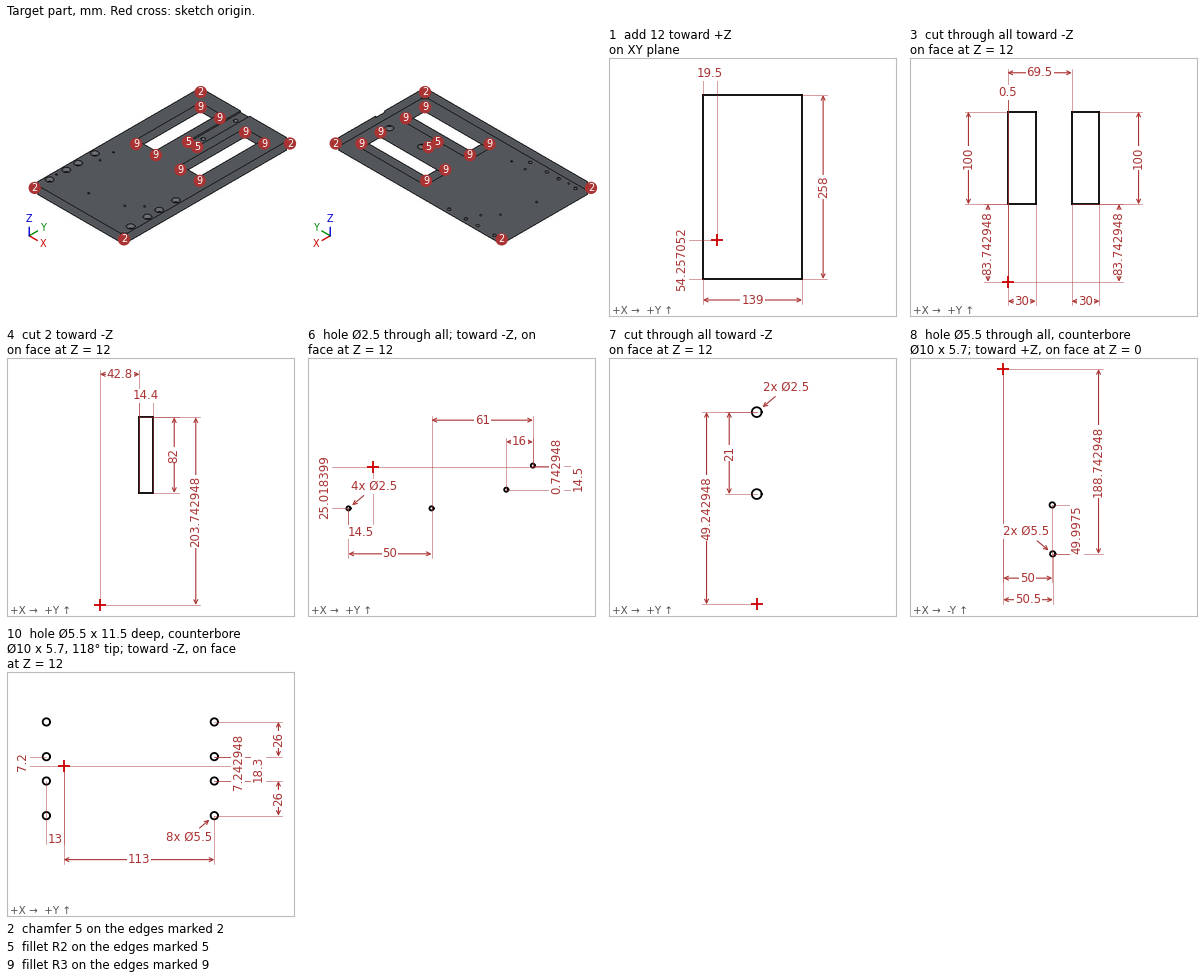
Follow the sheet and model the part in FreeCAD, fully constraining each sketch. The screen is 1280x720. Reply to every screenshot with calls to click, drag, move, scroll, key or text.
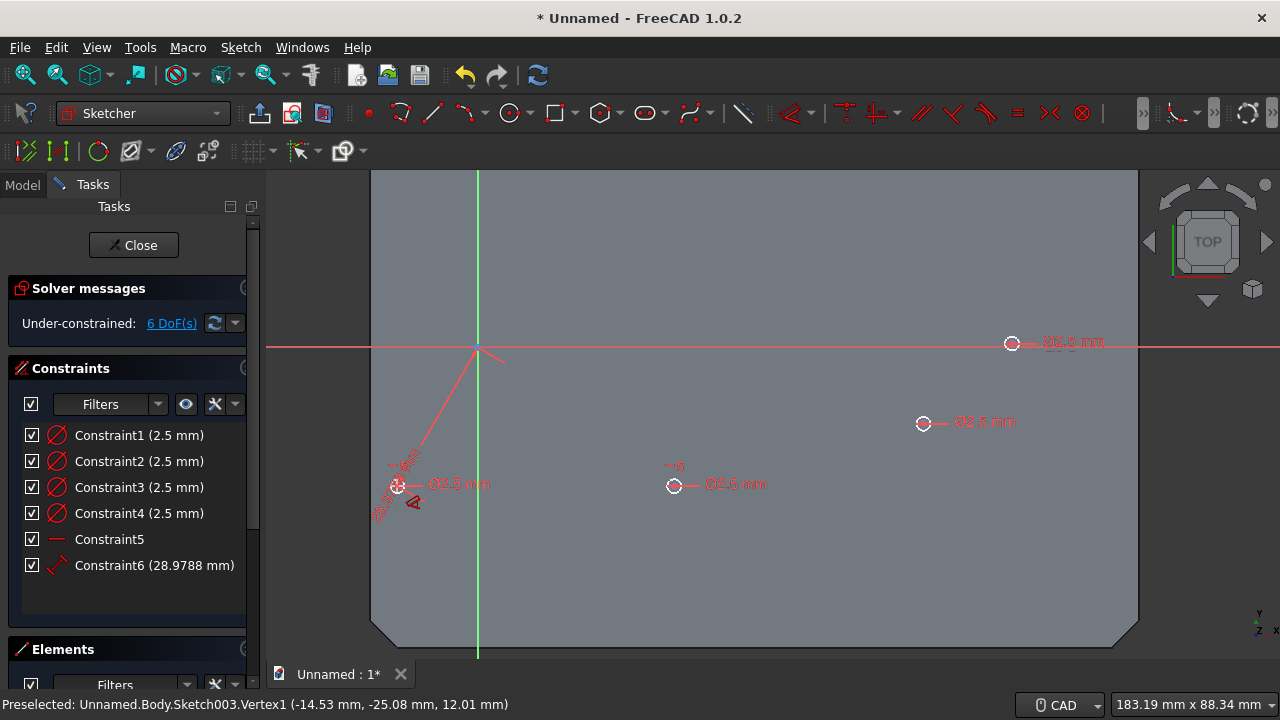
click(674, 486)
click(536, 520)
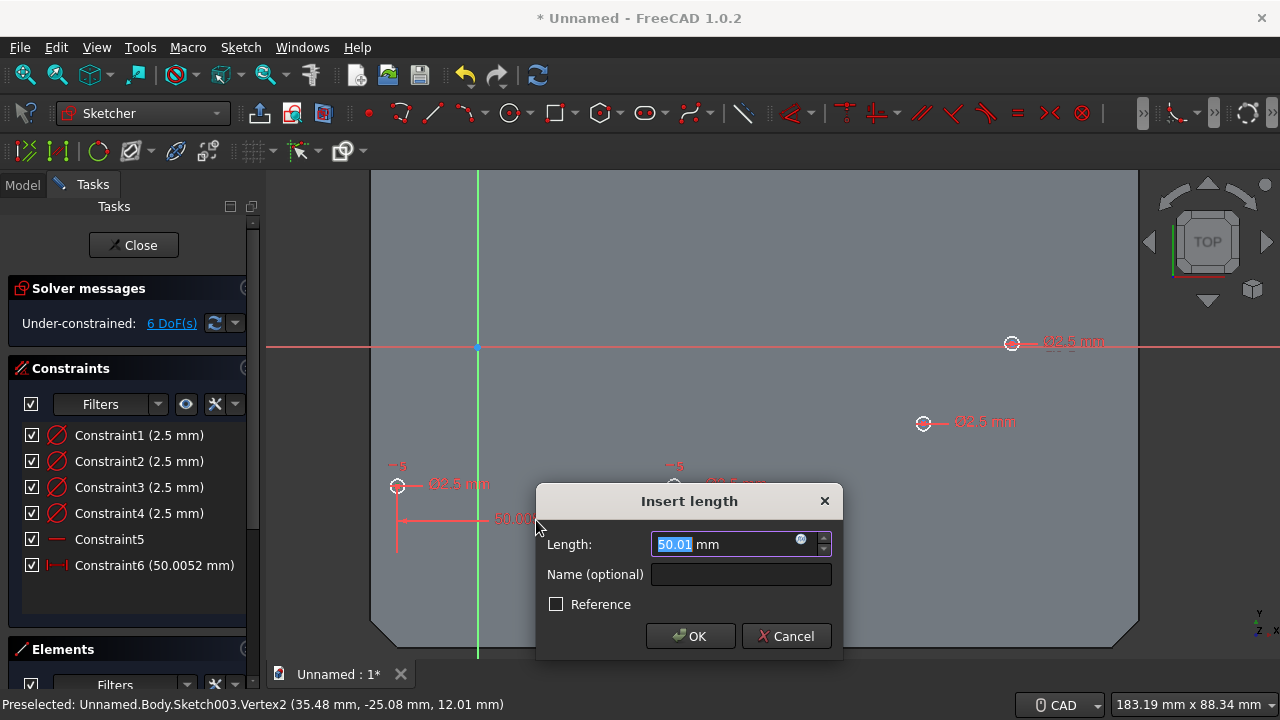
text(50)
key(Return)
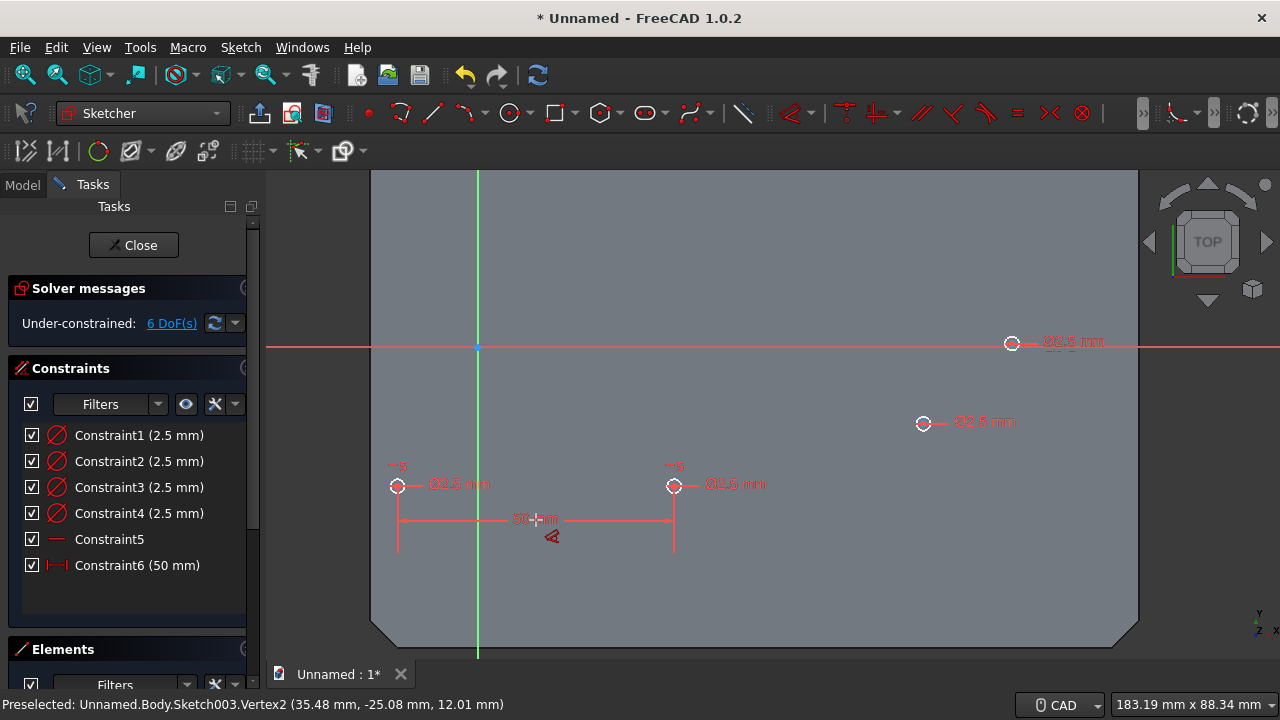
click(674, 486)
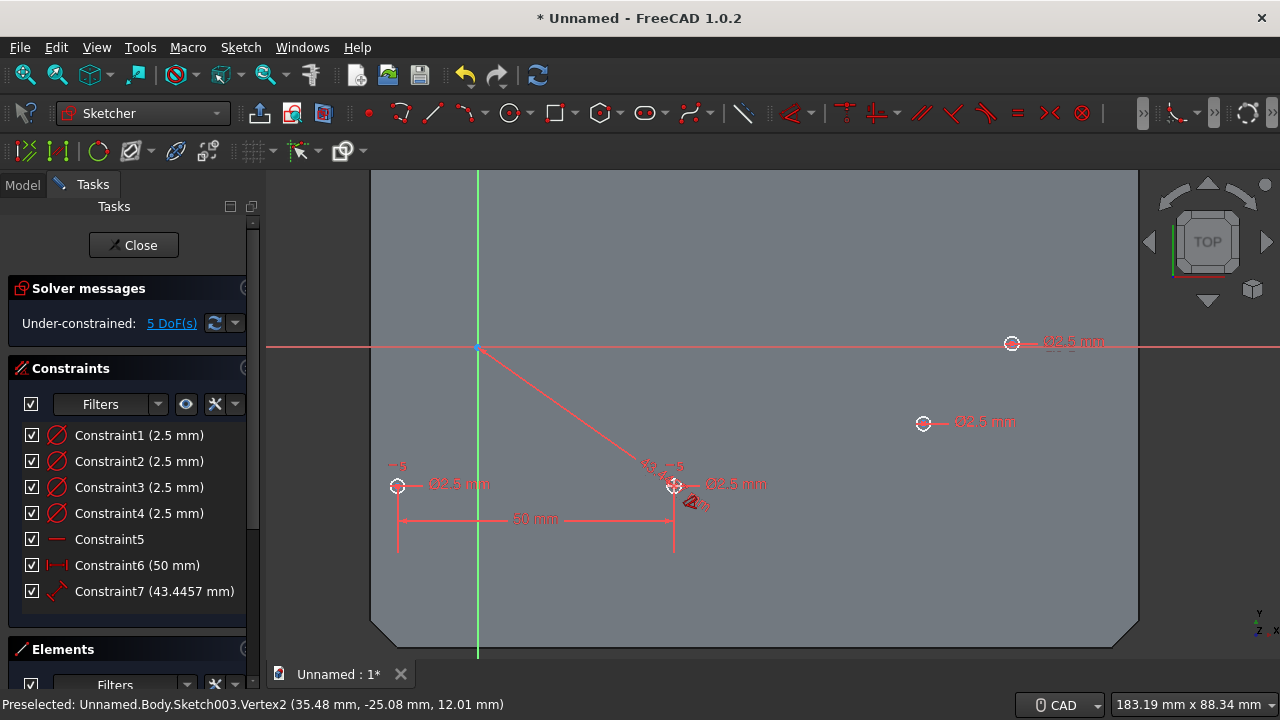
click(1012, 344)
click(843, 520)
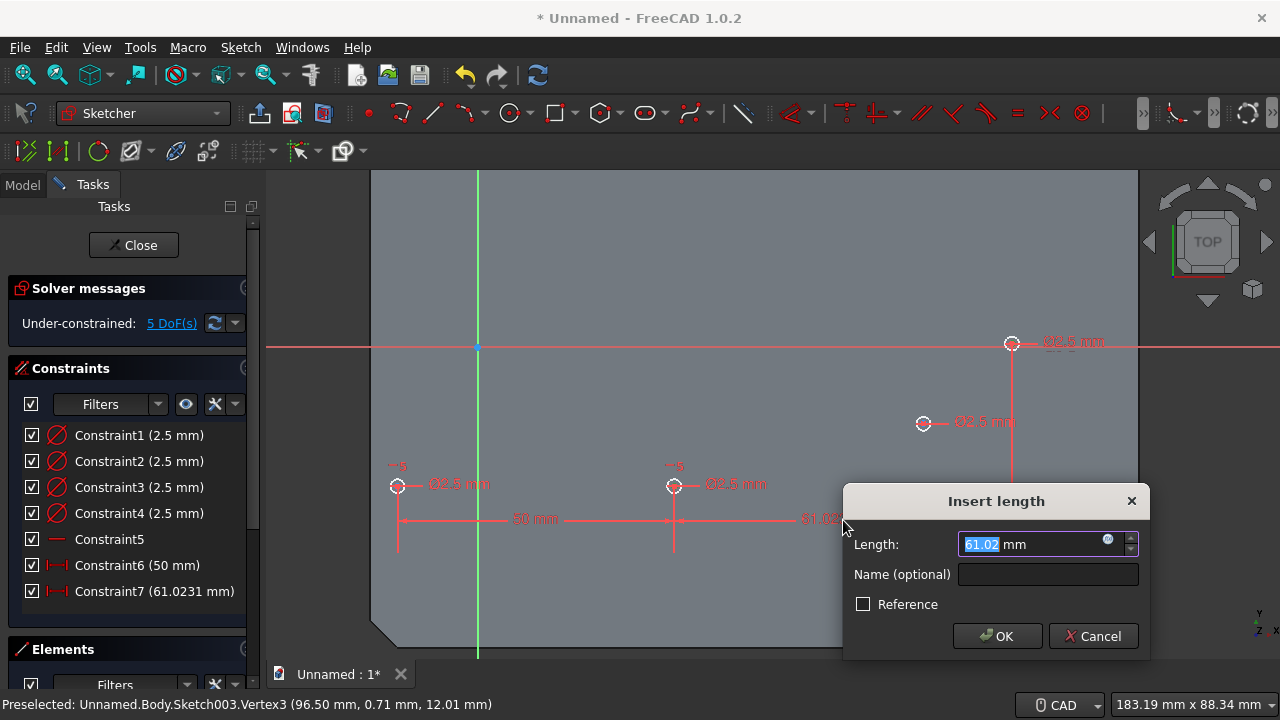
text(61)
key(Return)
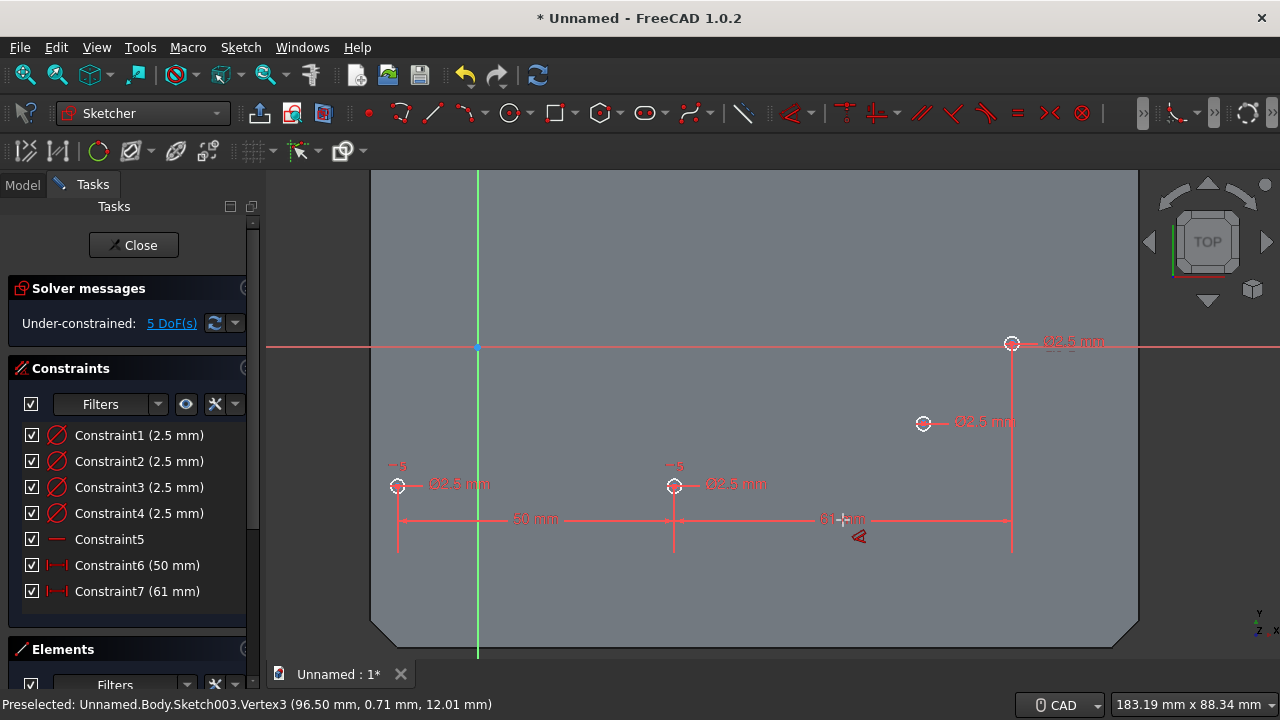
click(1012, 344)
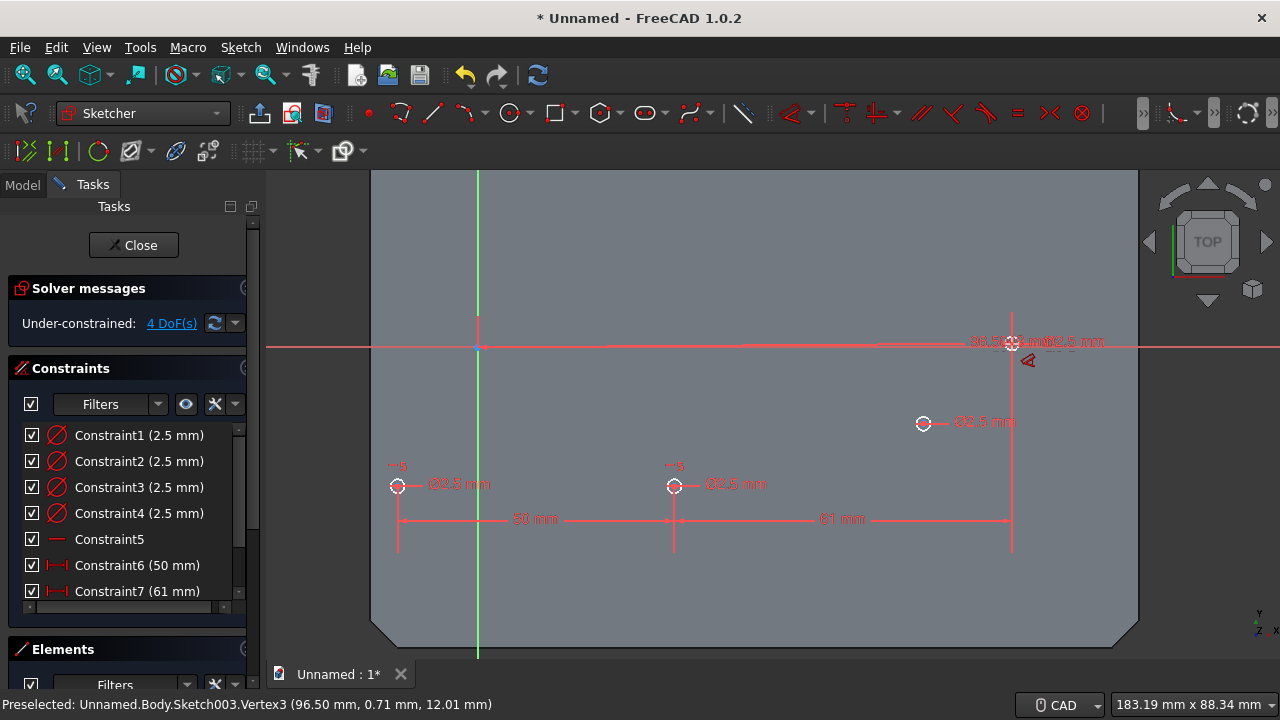
click(923, 424)
click(968, 310)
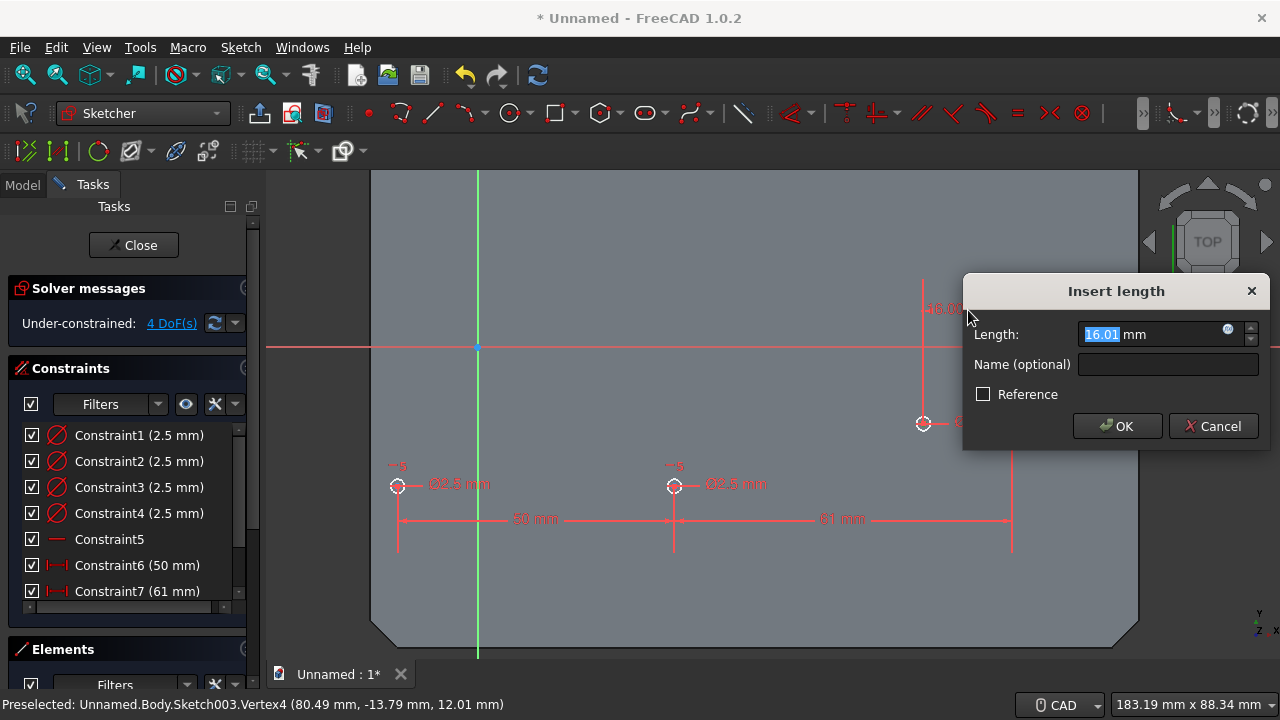
text(16)
key(Return)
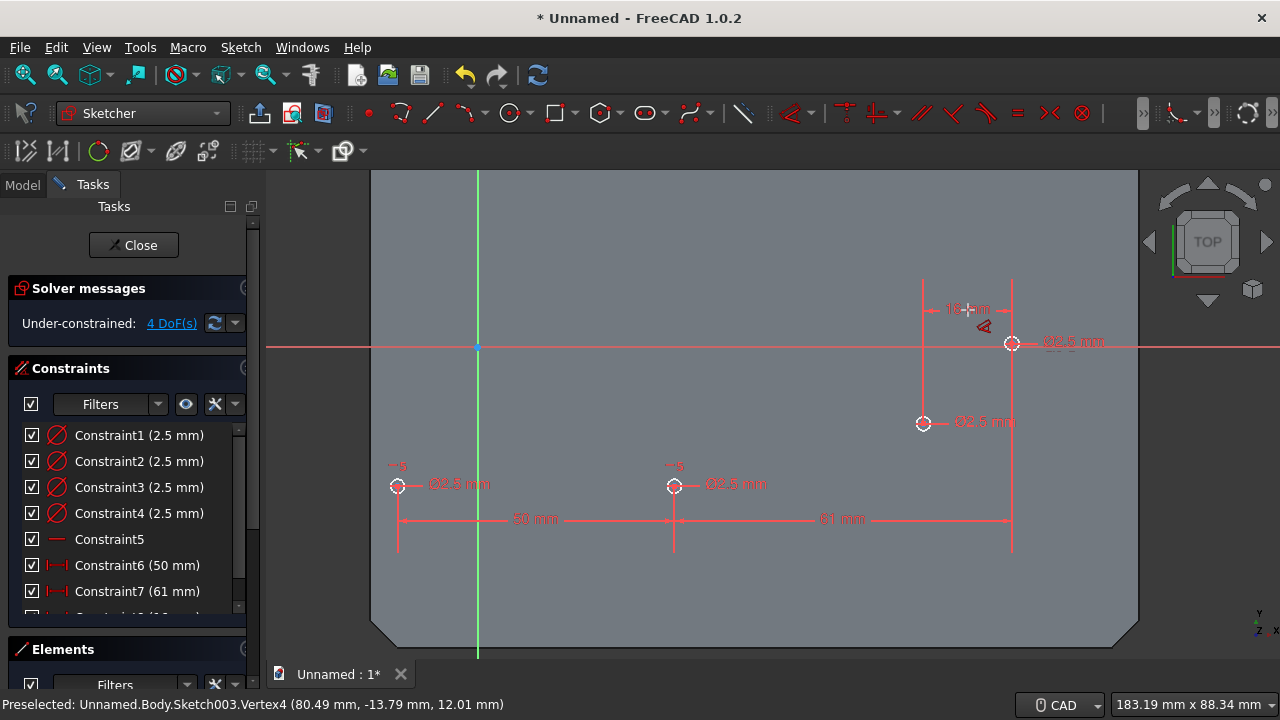
click(398, 486)
click(438, 520)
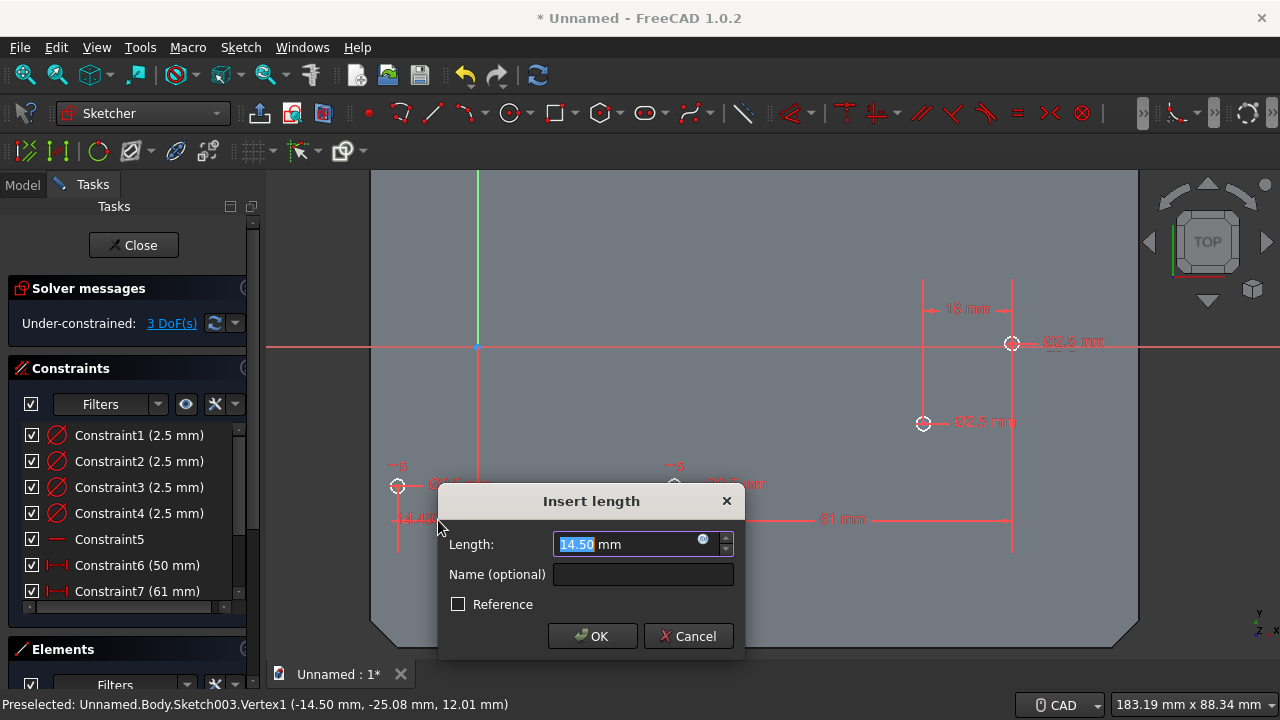
text(14.5)
key(Return)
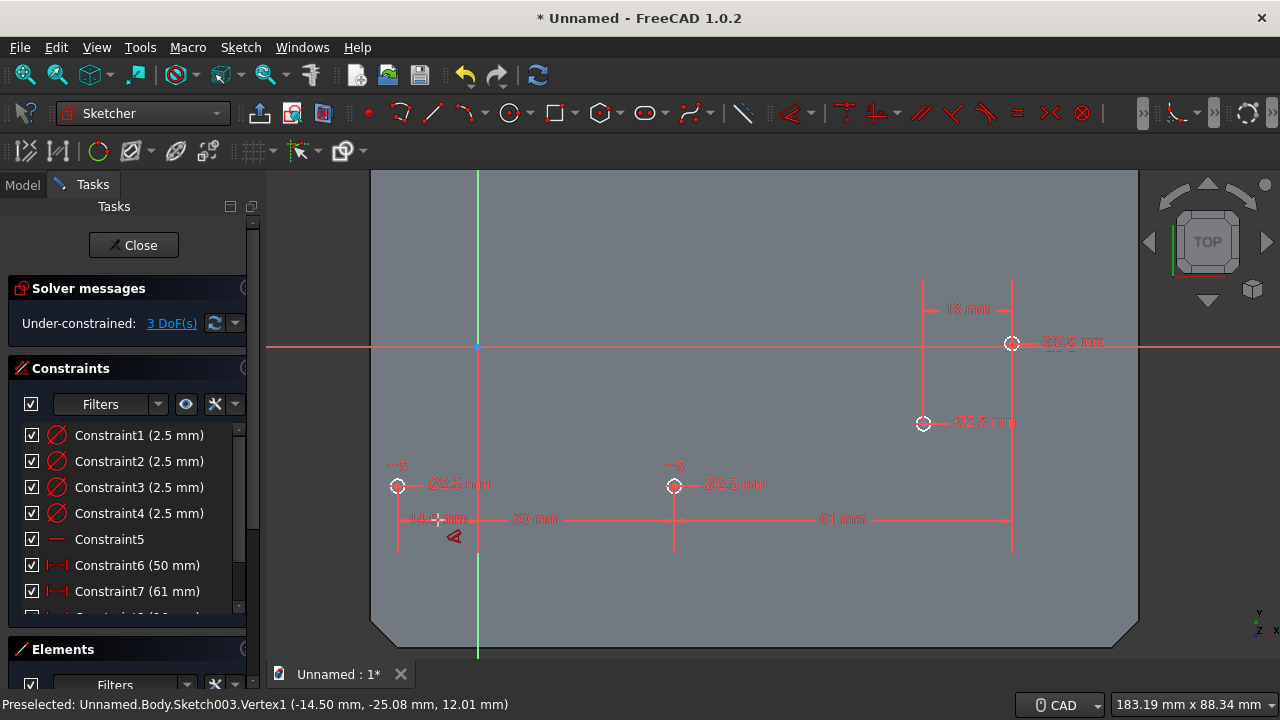
click(1012, 344)